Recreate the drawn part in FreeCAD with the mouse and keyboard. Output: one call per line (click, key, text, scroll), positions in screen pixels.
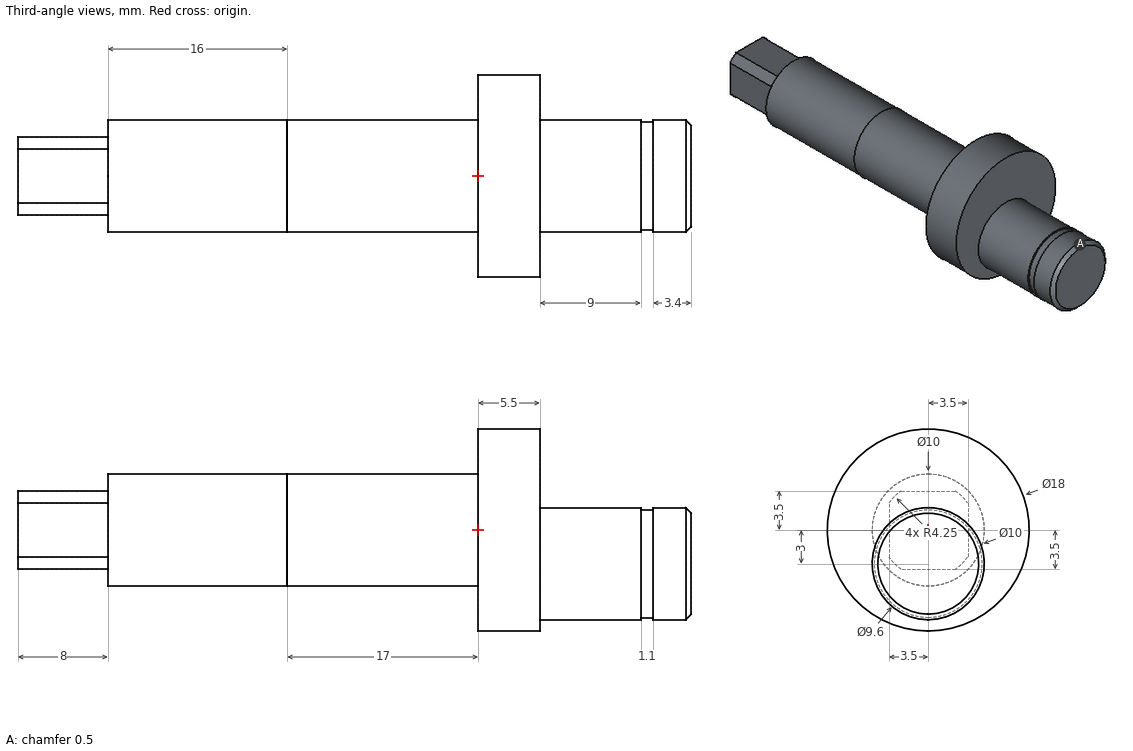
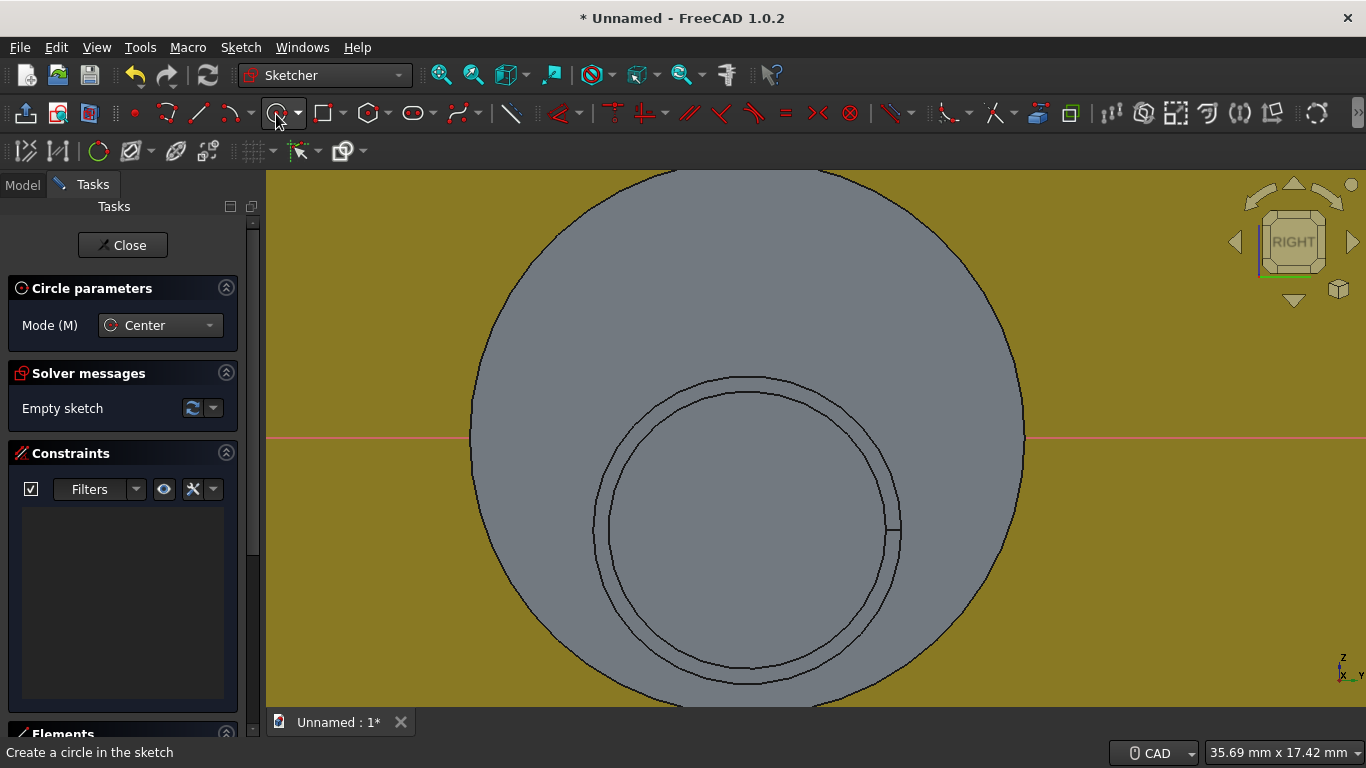
click(747, 438)
click(856, 329)
key(Escape)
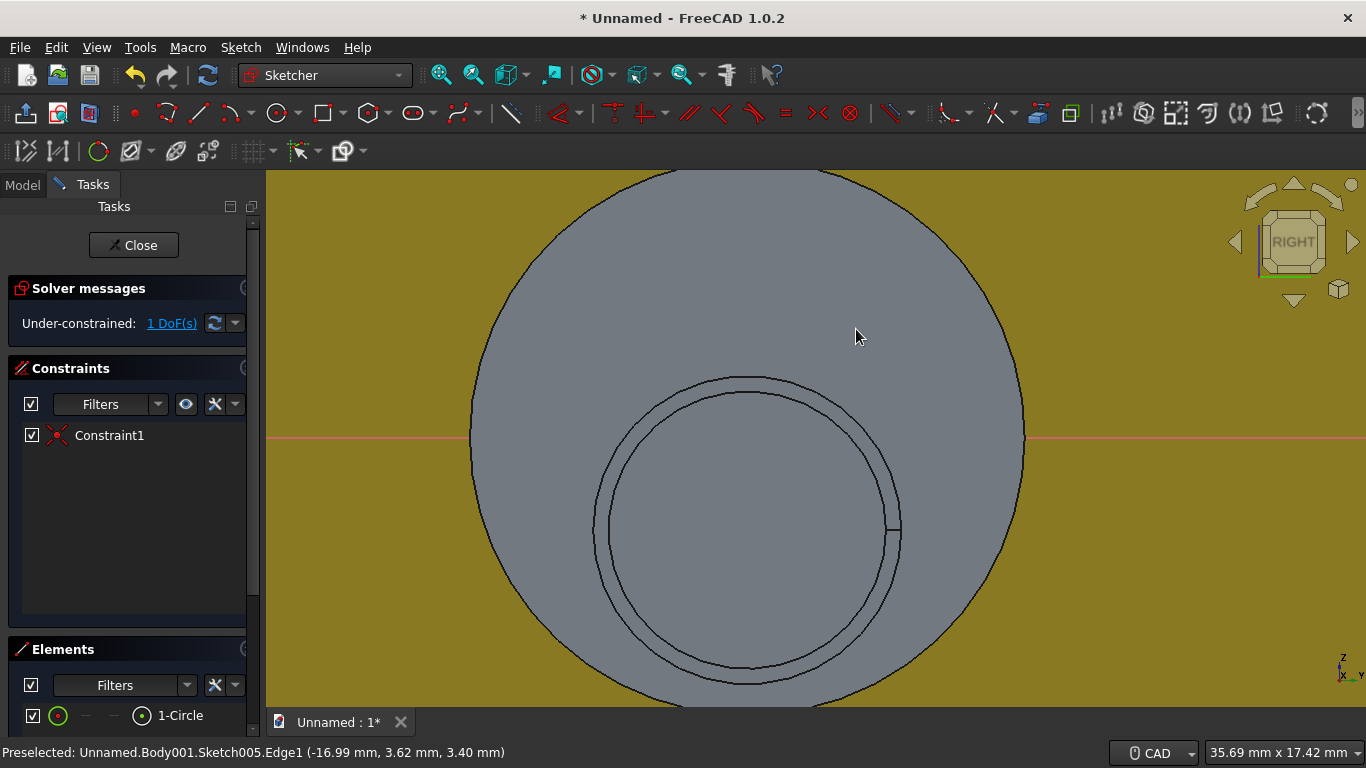
key(d)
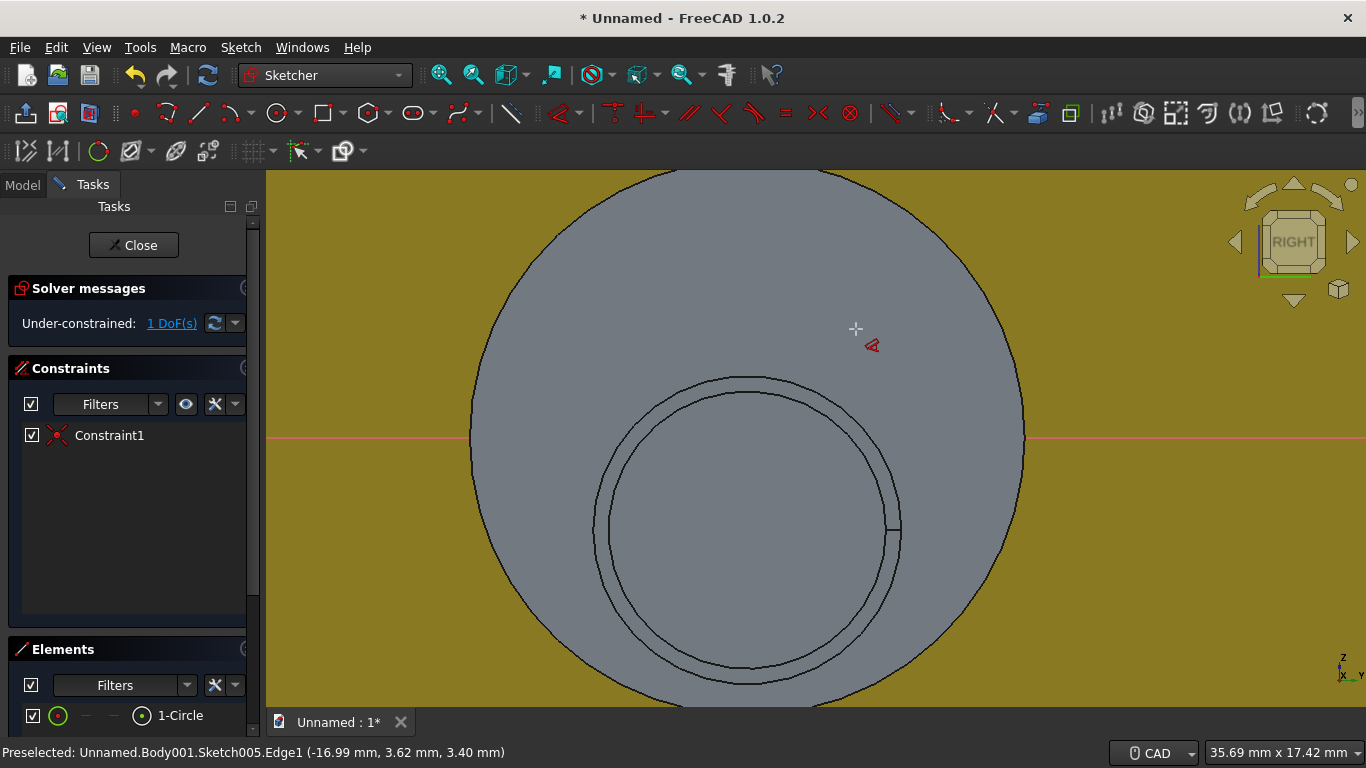
click(855, 329)
click(878, 306)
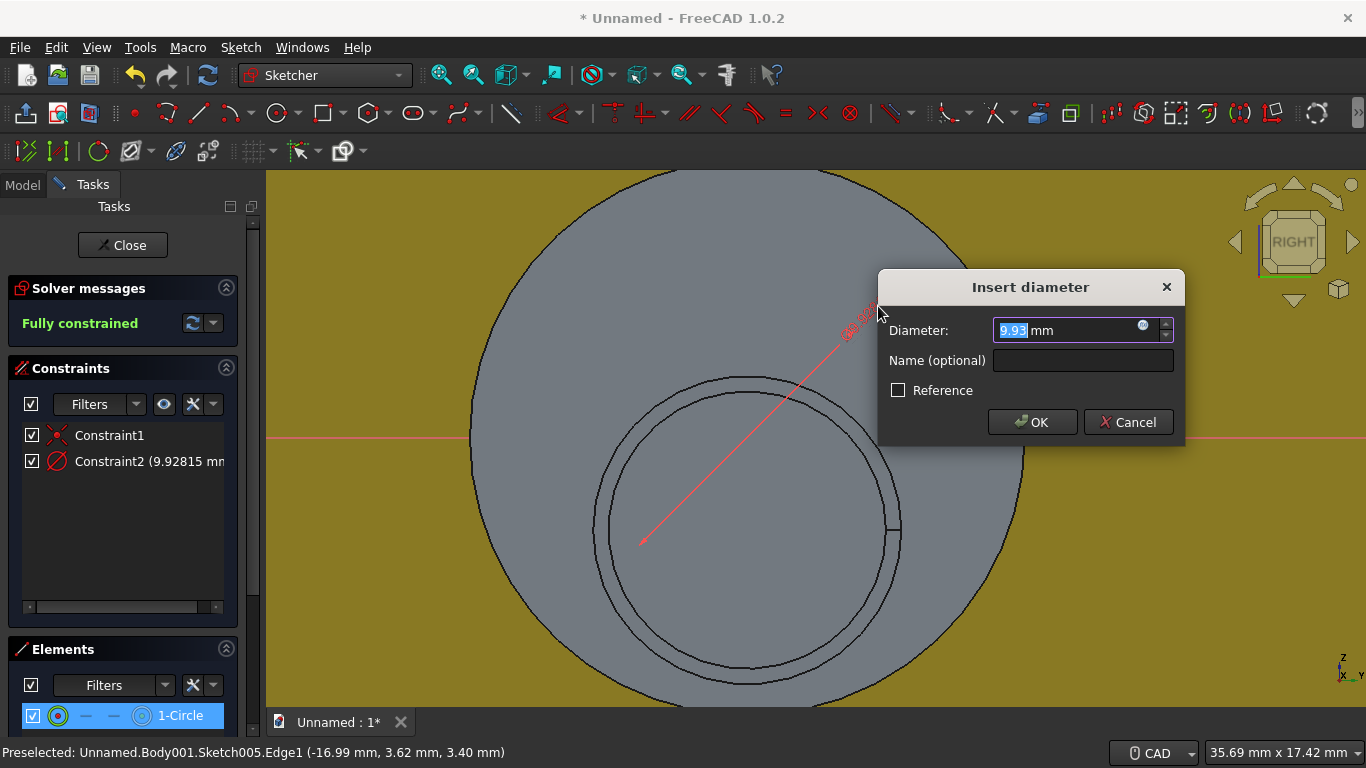
text(10)
key(Return)
key(Escape)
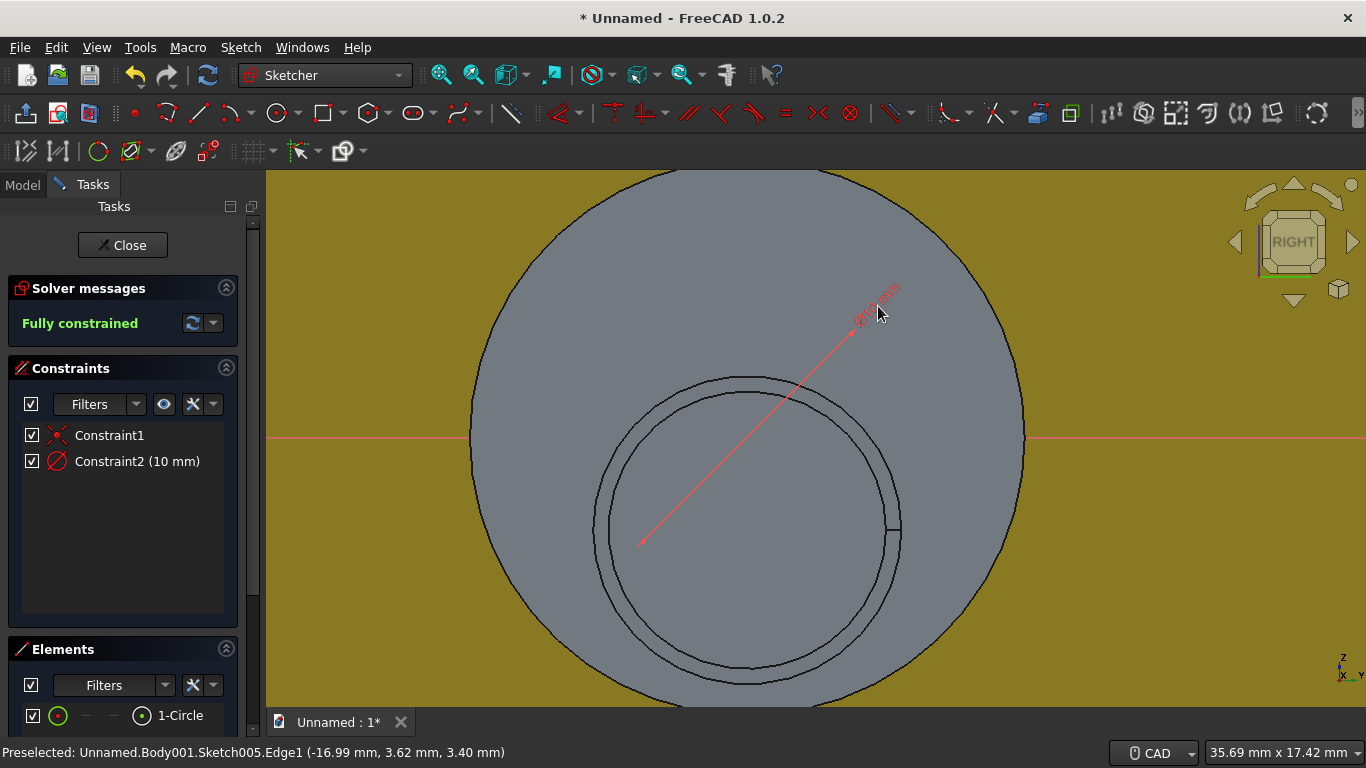
click(123, 245)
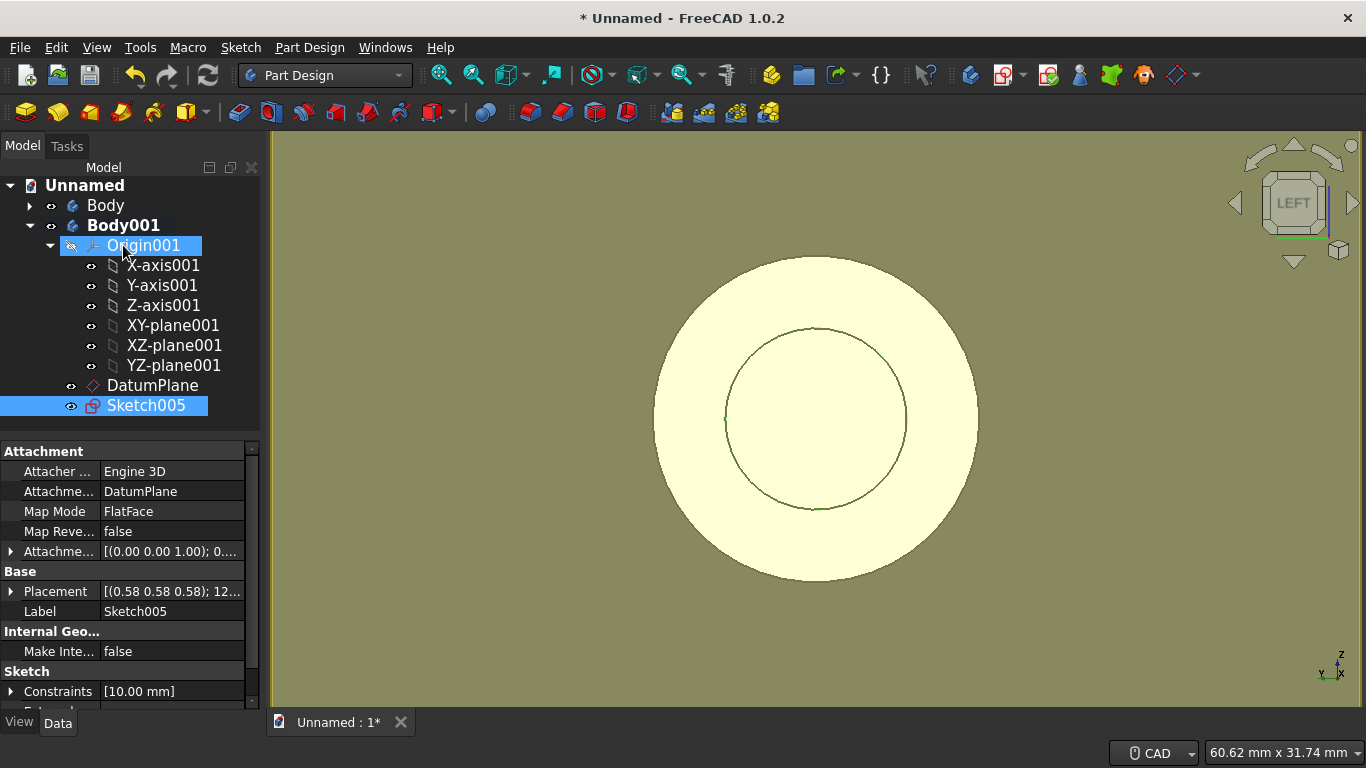
click(26, 112)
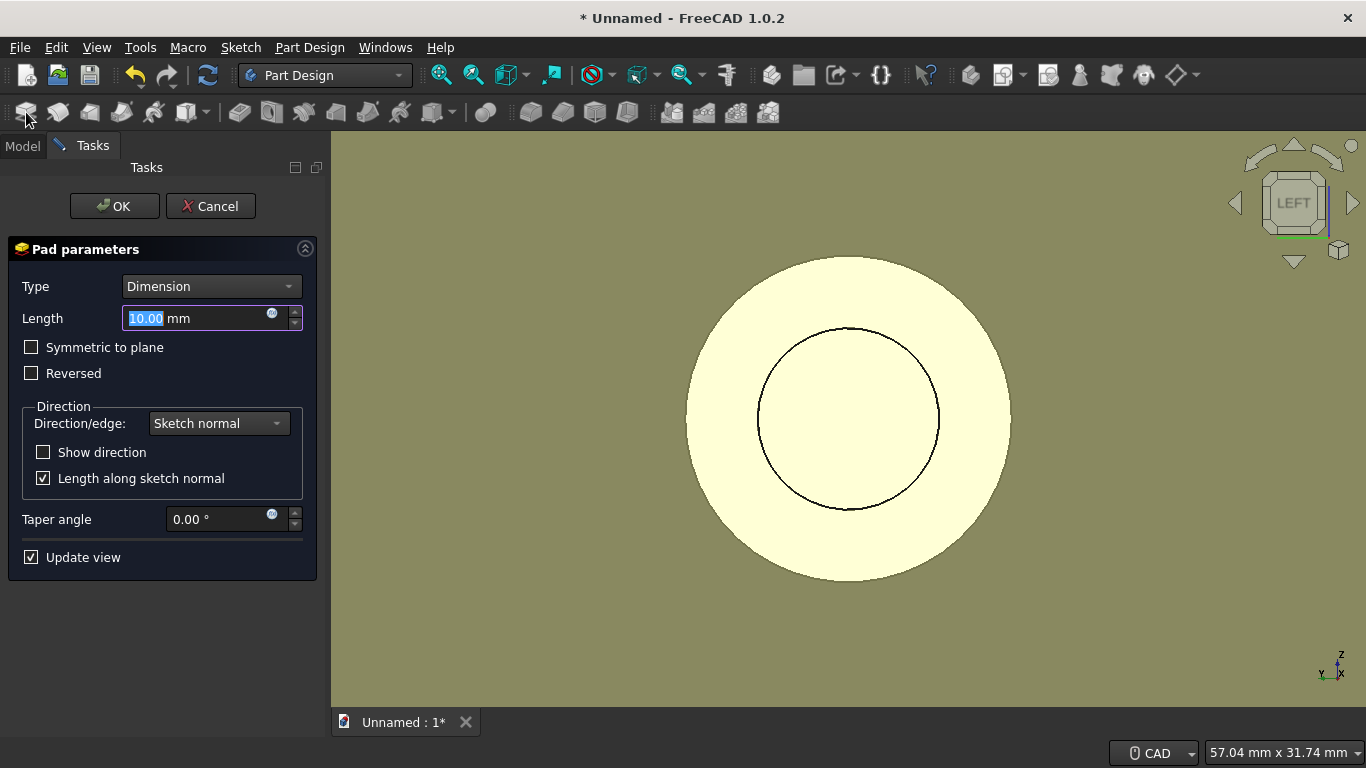
text(16)
key(Tab)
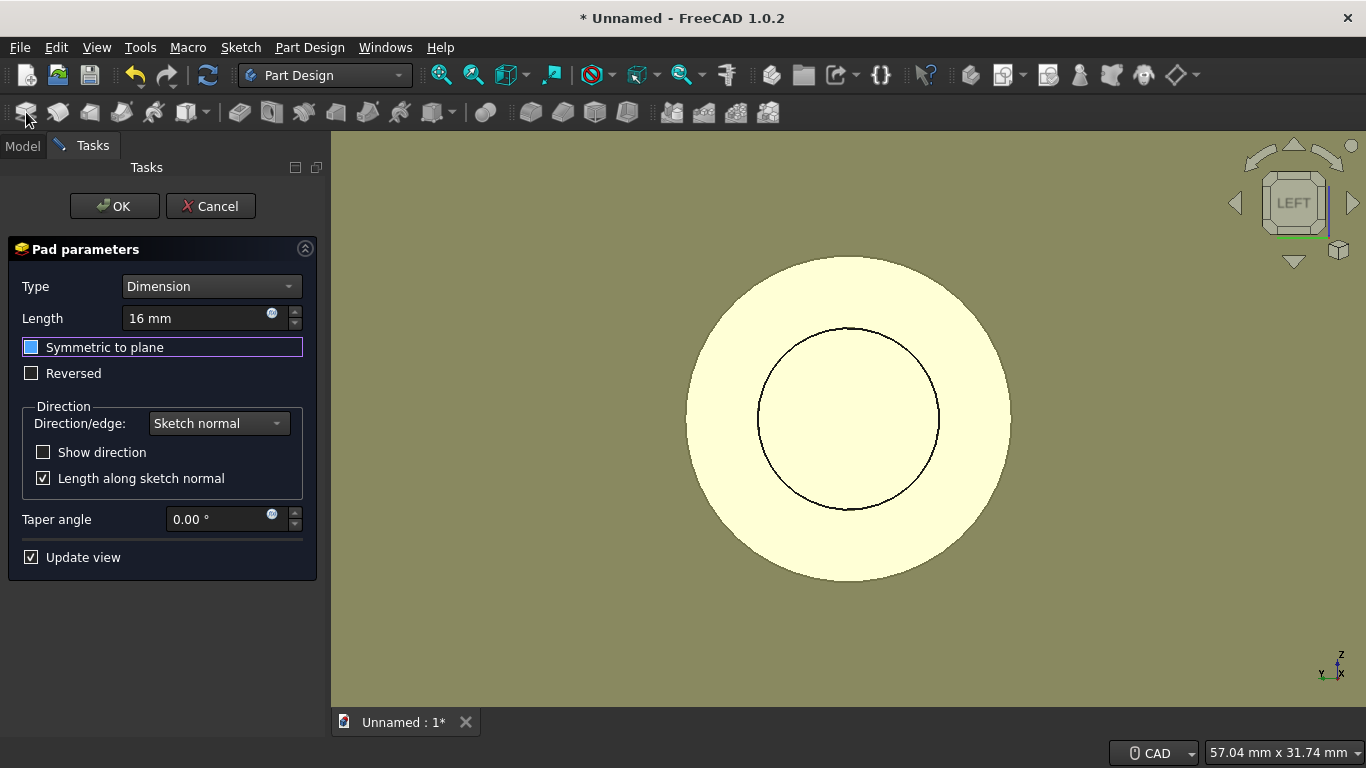
click(30, 373)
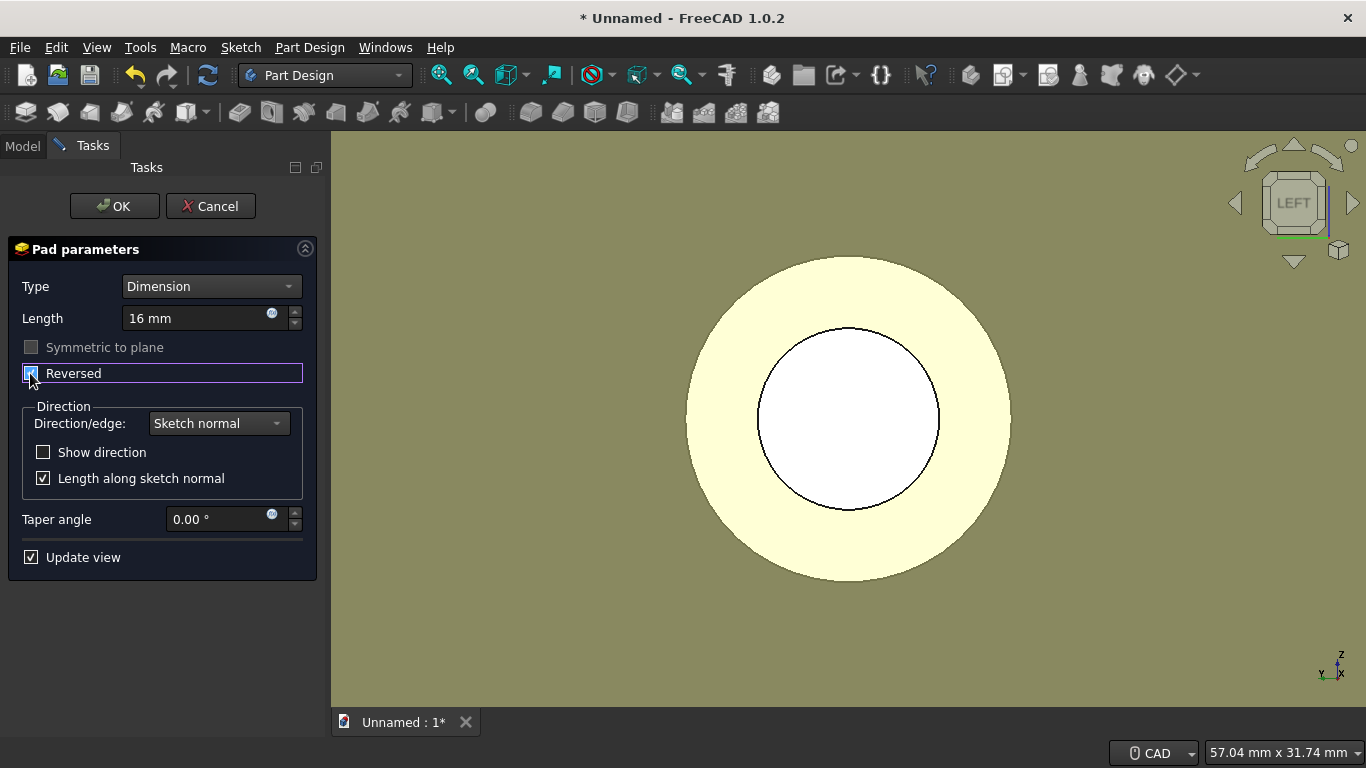
click(115, 206)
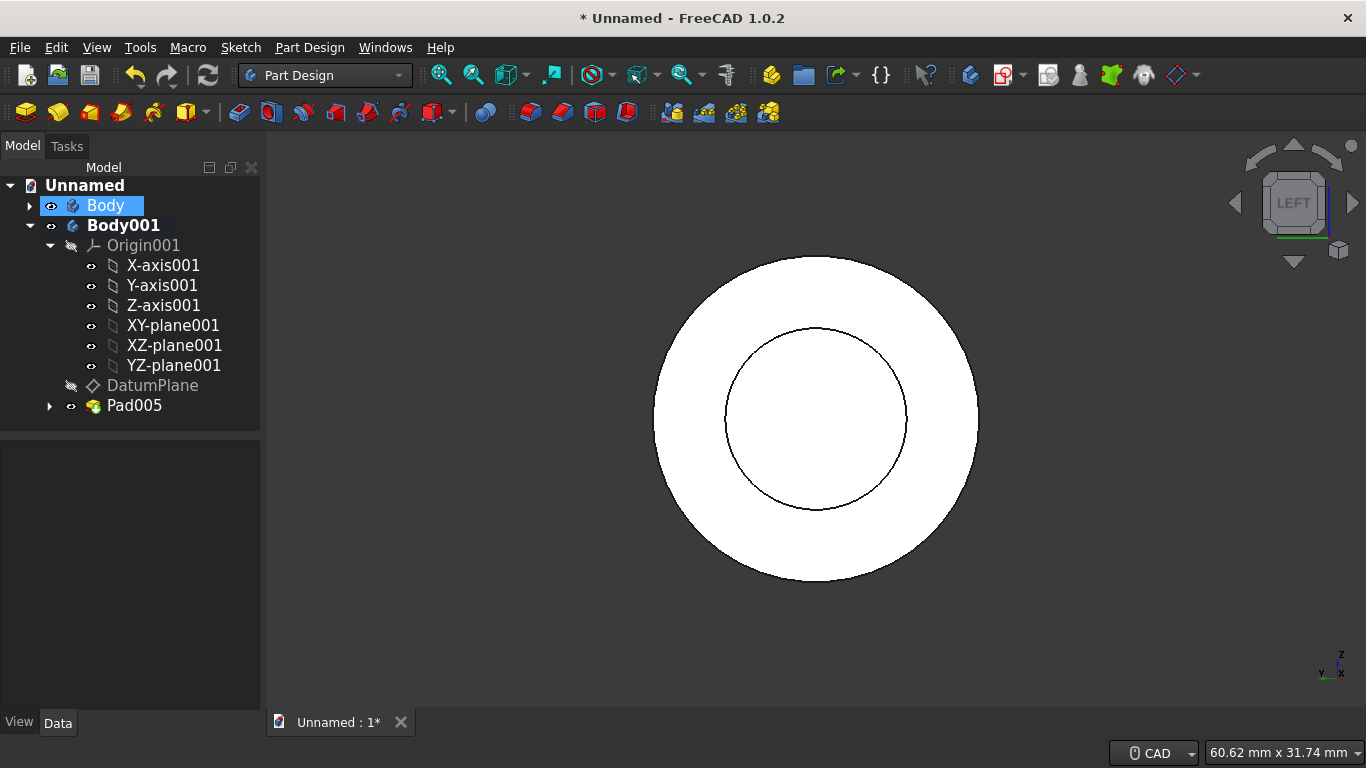
click(442, 76)